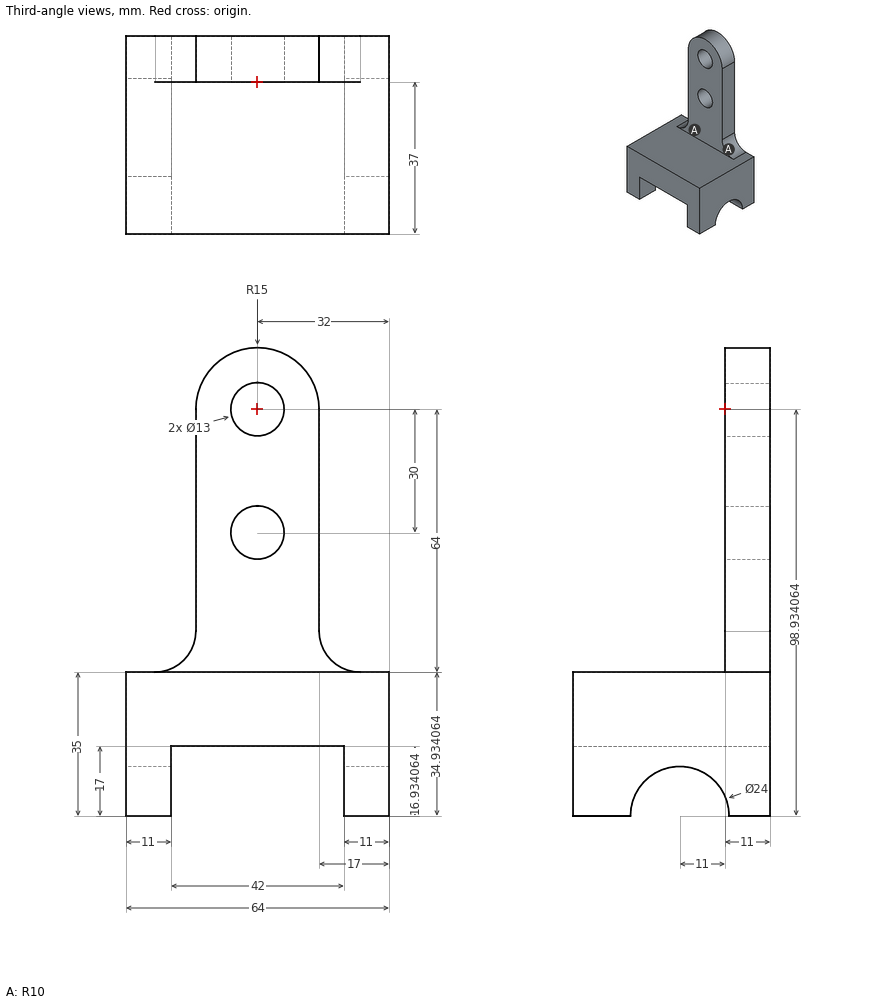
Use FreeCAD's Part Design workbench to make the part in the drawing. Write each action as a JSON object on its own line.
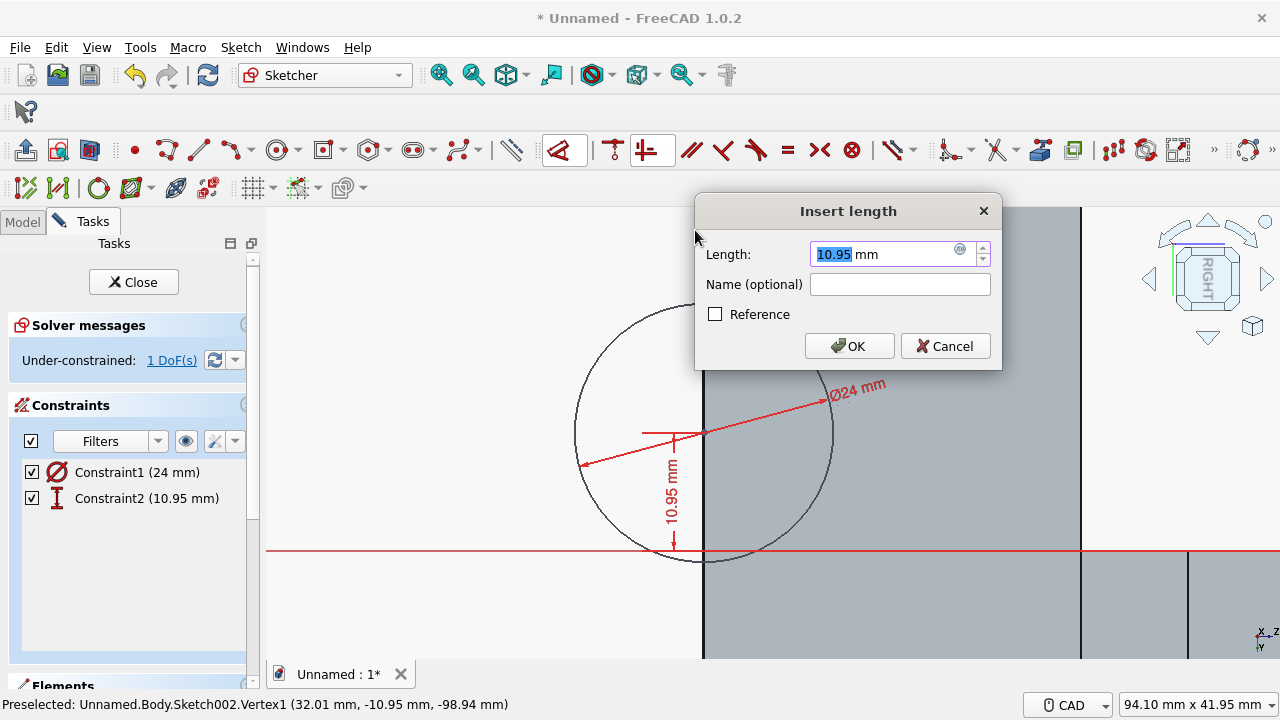
{"action": "type", "text": "11"}
{"action": "key", "text": "Return"}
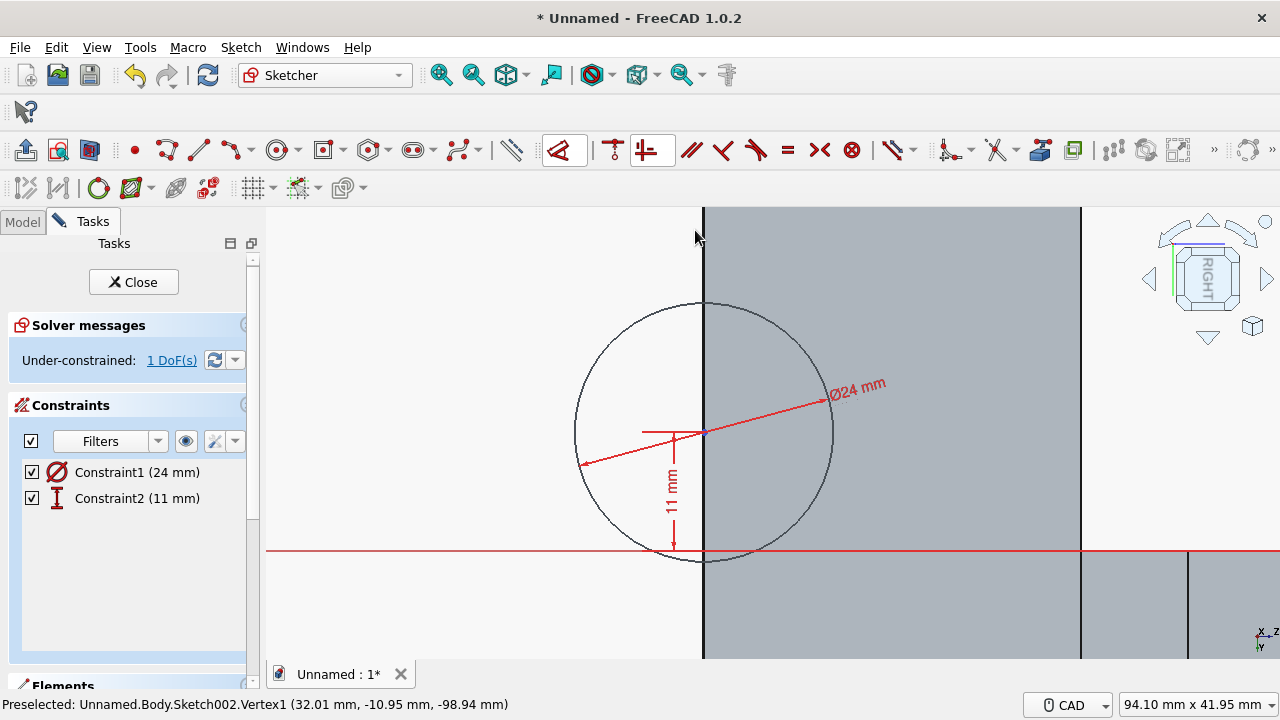
{"action": "left_click", "coordinate": [704, 432]}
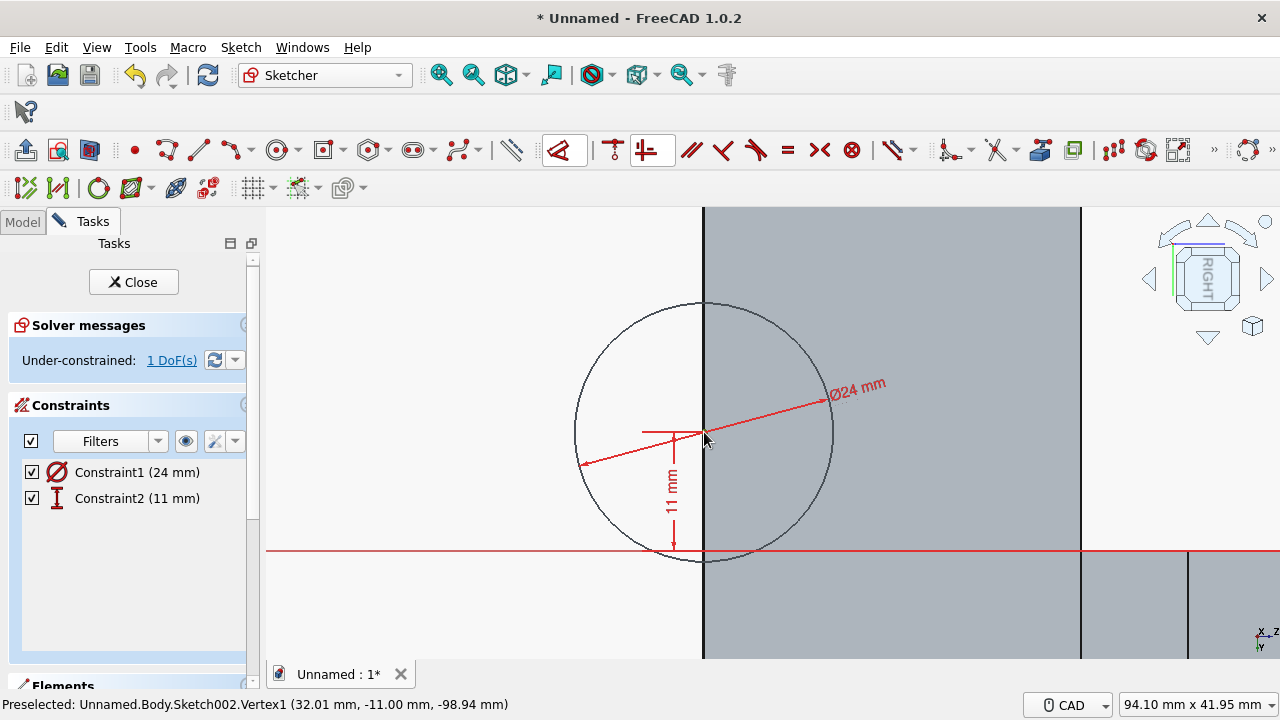
{"action": "key", "text": "l"}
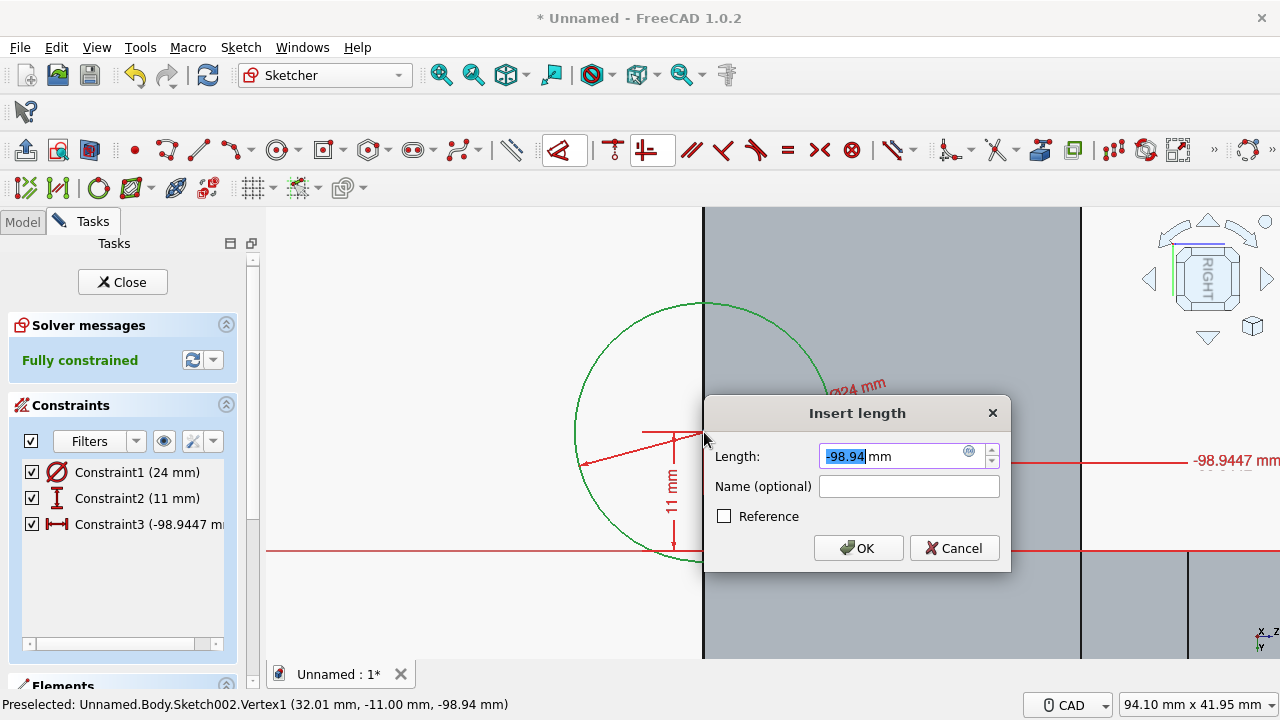
{"action": "type", "text": "-98.934064"}
{"action": "key", "text": "Return"}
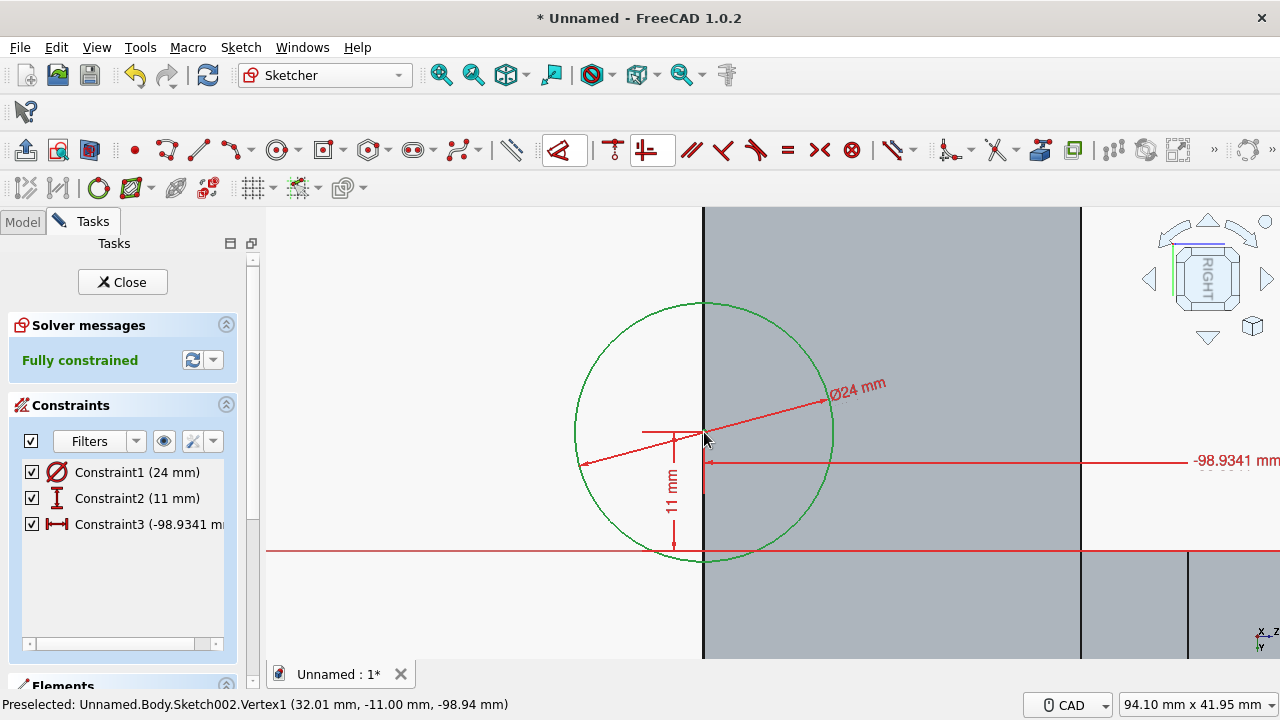
{"action": "left_click", "coordinate": [123, 282]}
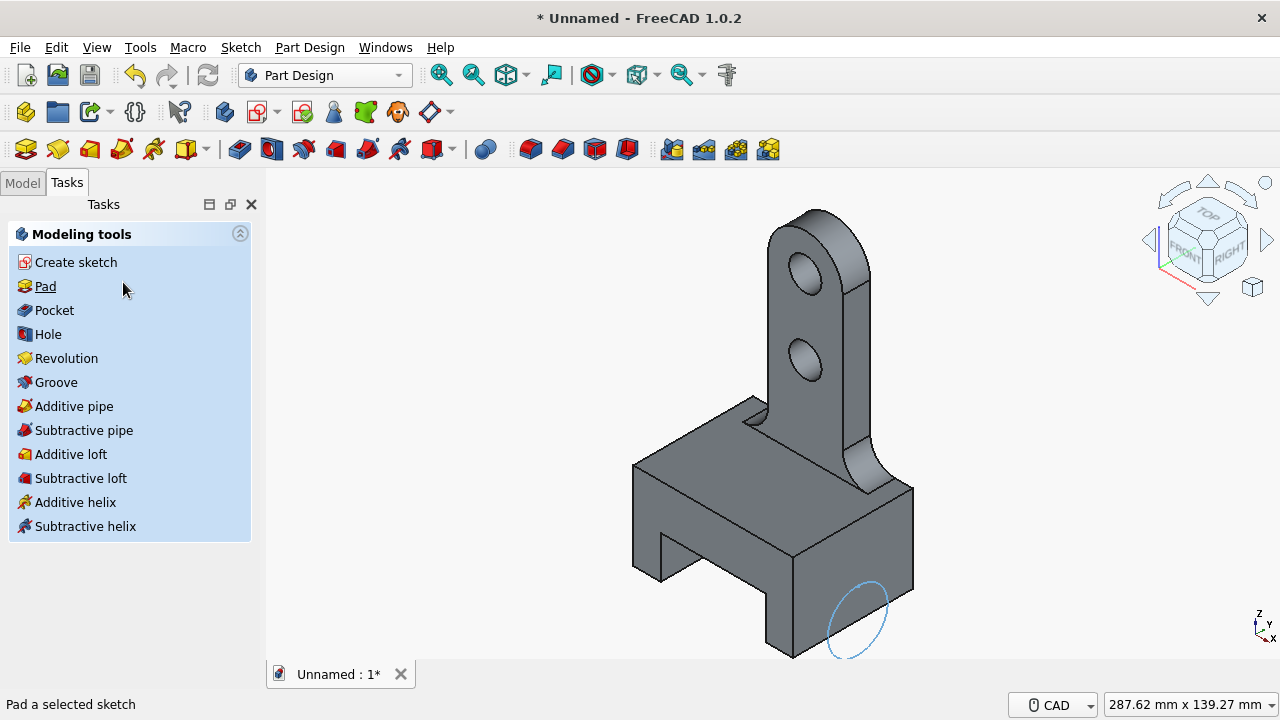
{"action": "left_click", "coordinate": [240, 150]}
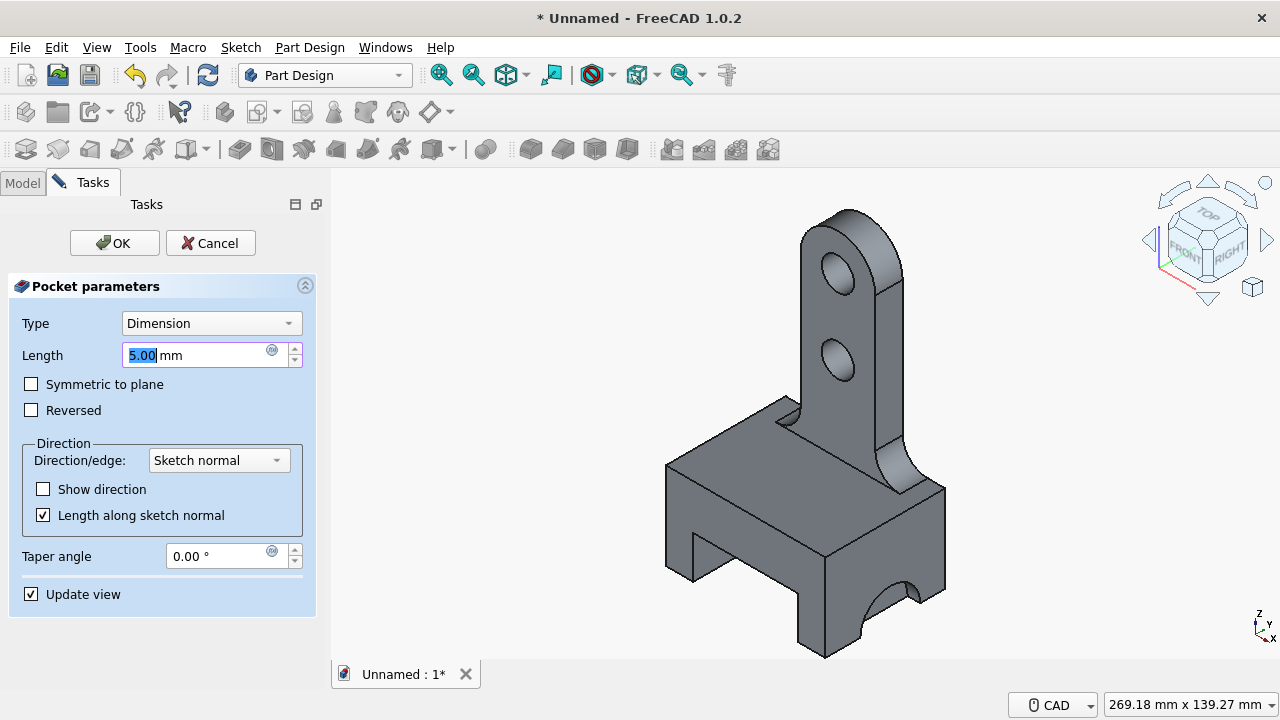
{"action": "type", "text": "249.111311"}
{"action": "key", "text": "Tab"}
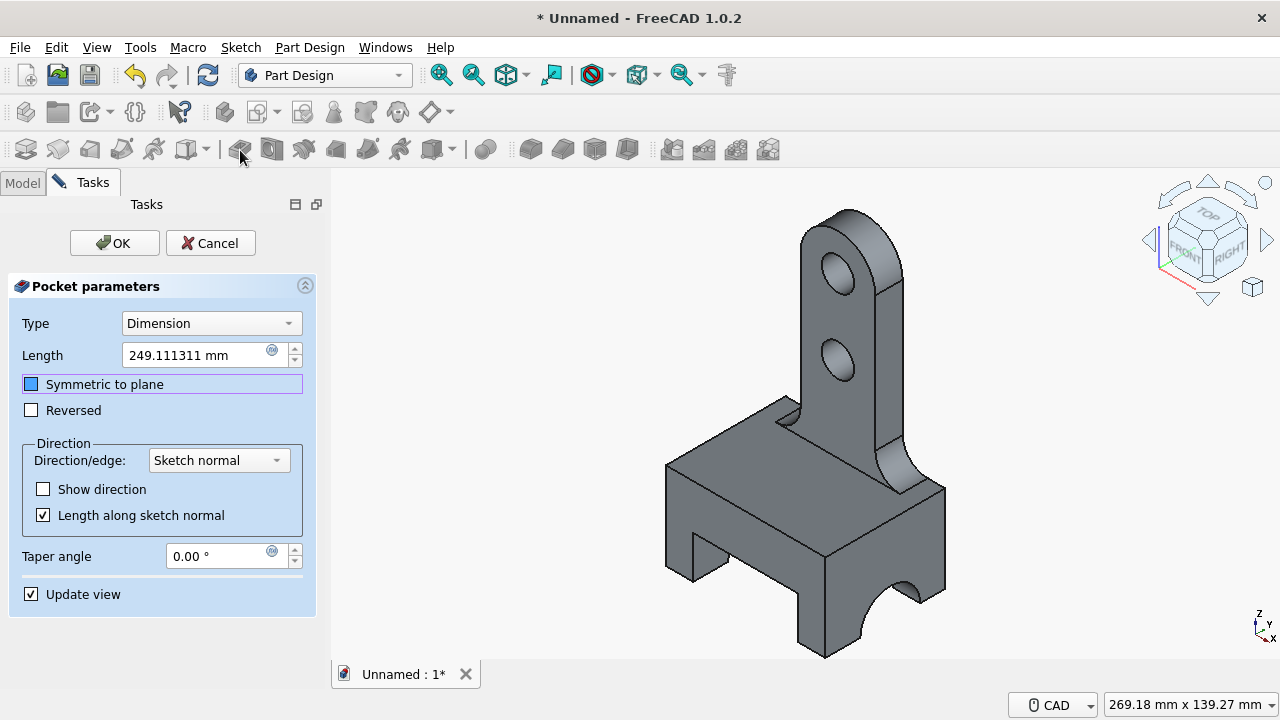
{"action": "left_click", "coordinate": [30, 384]}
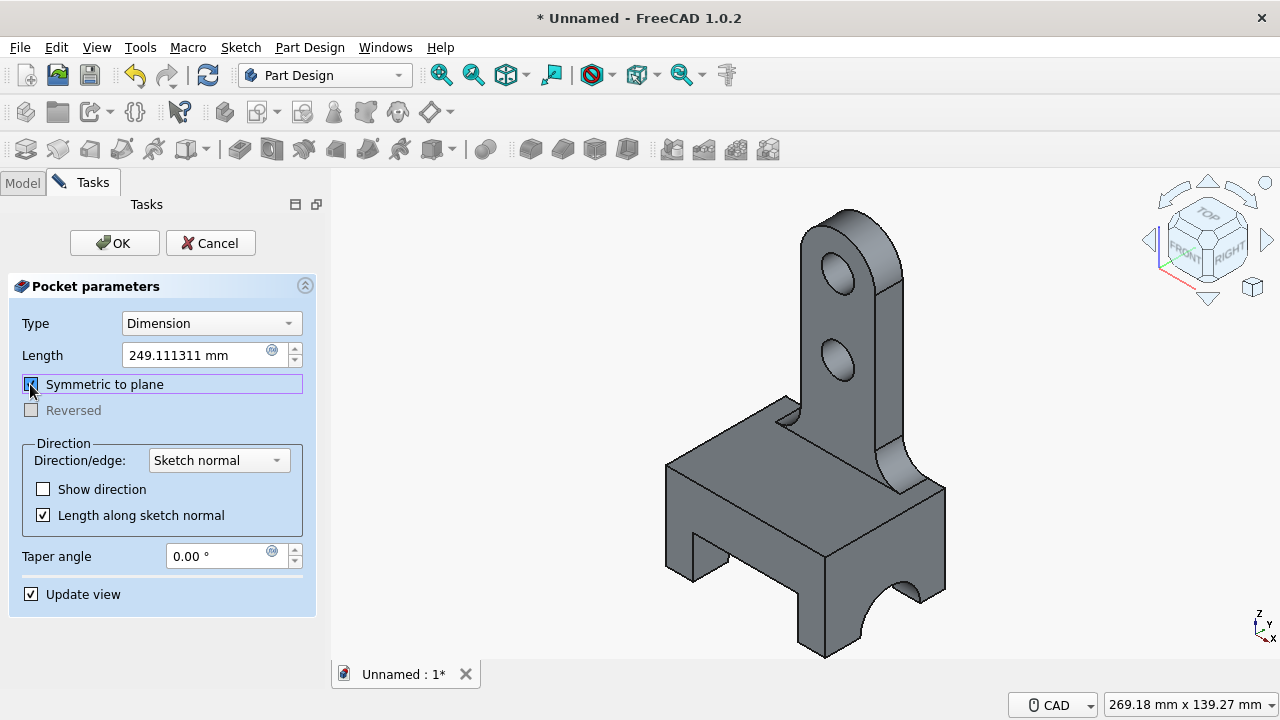
{"action": "left_click", "coordinate": [115, 243]}